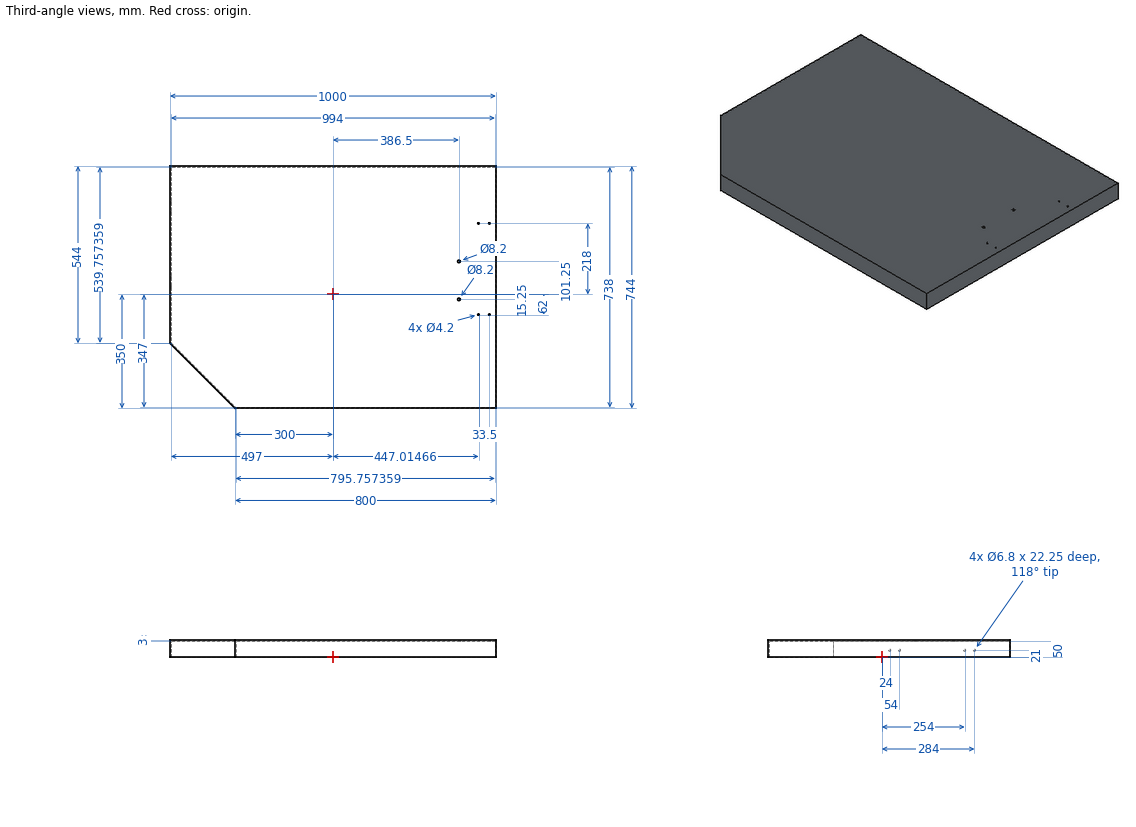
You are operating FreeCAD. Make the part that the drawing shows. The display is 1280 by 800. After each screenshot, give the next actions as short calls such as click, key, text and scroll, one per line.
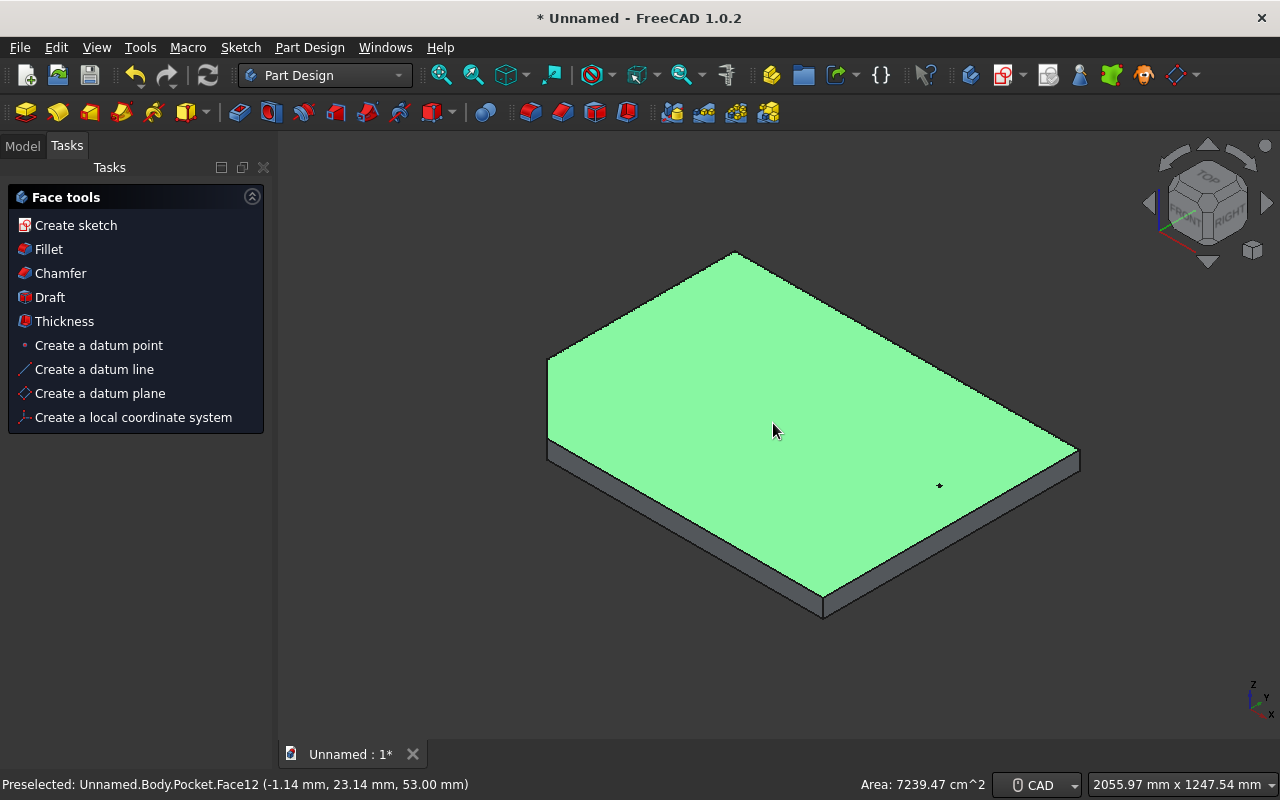
click(1004, 76)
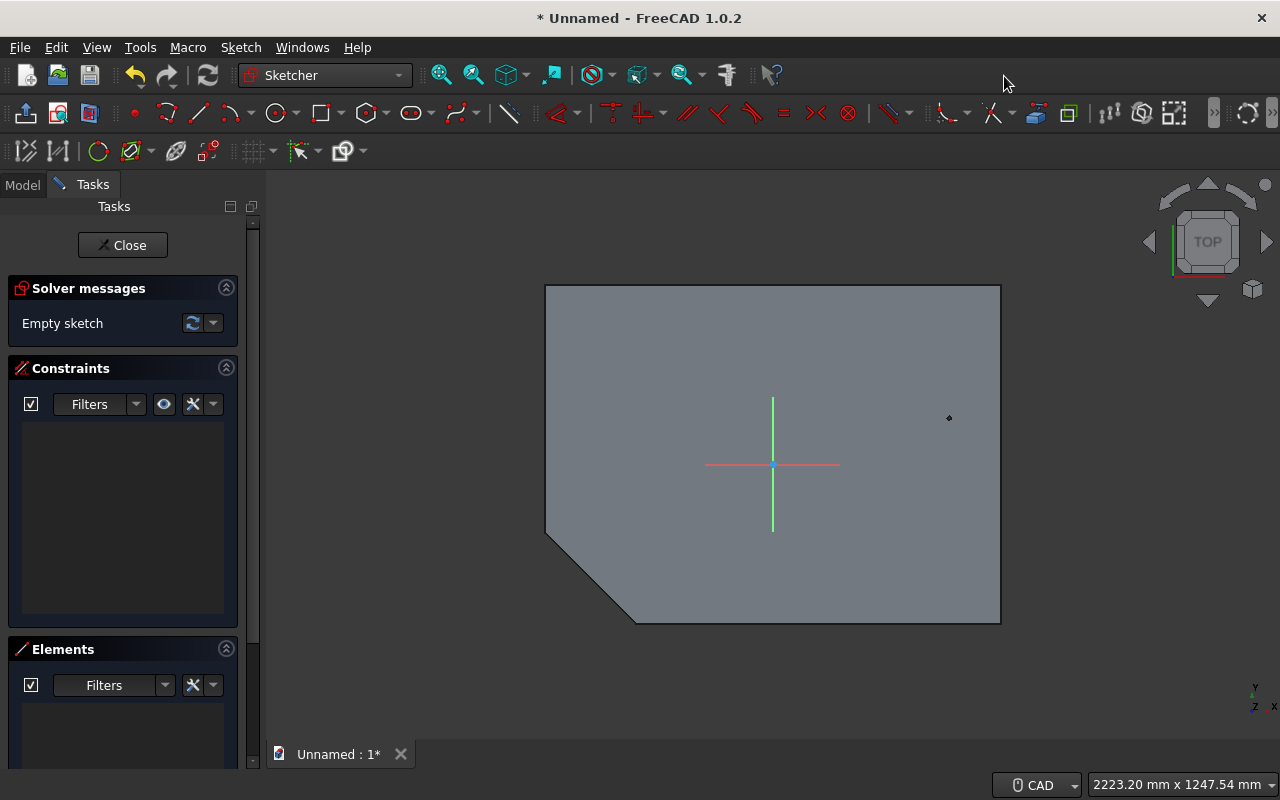
scroll(962, 472, up, 15)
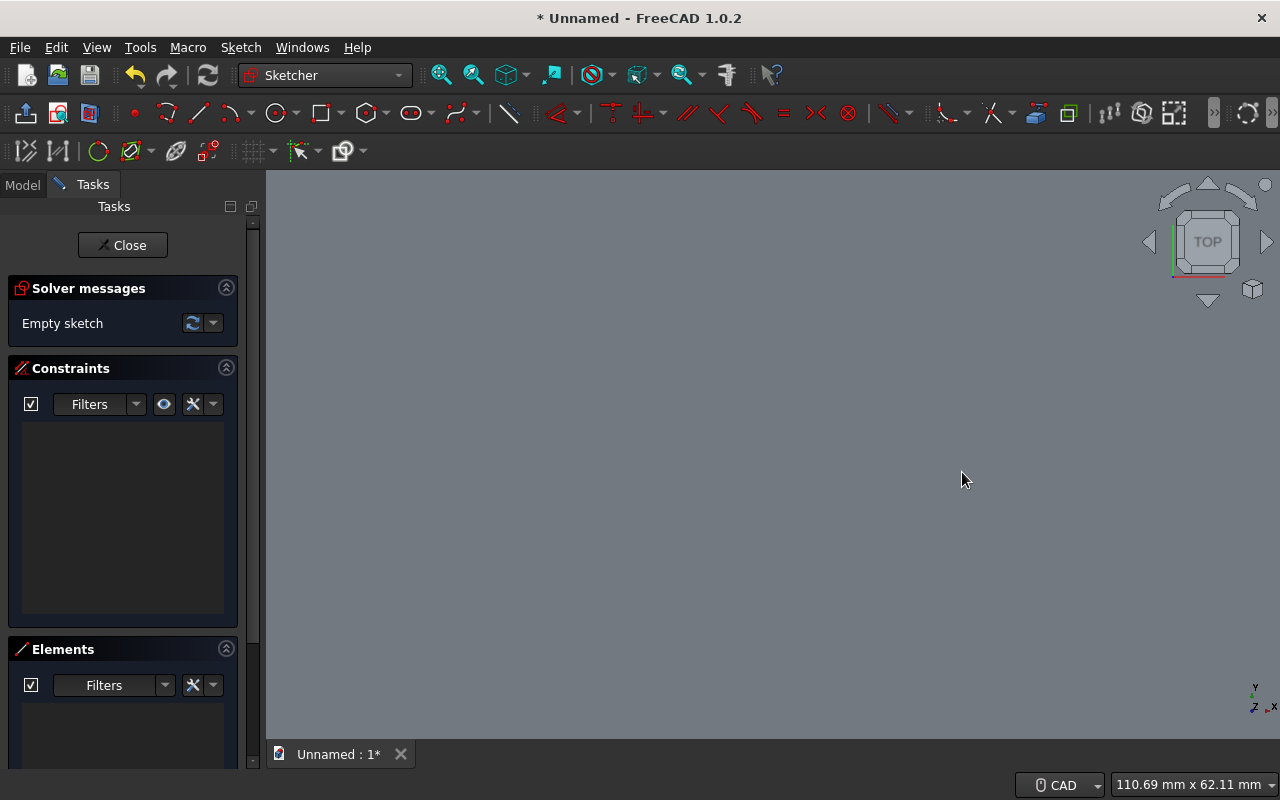
scroll(691, 451, up, 8)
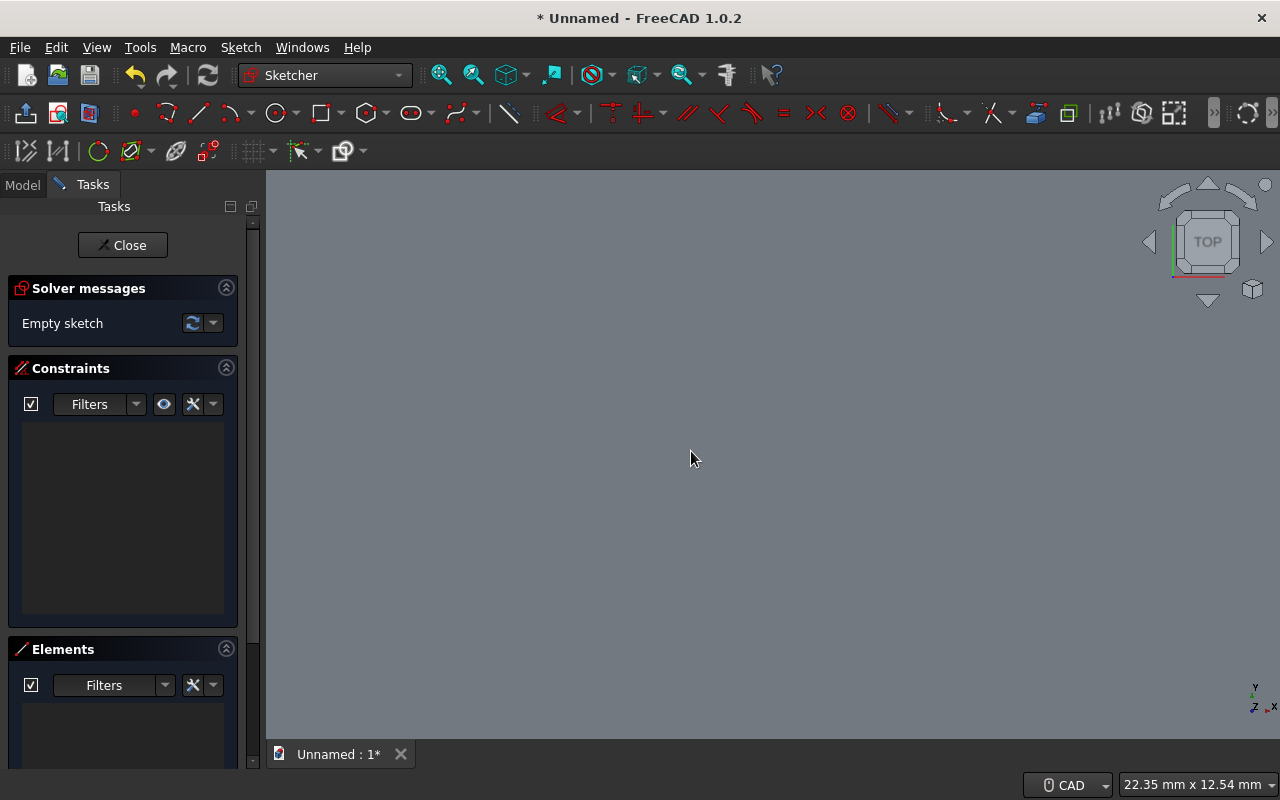
click(276, 114)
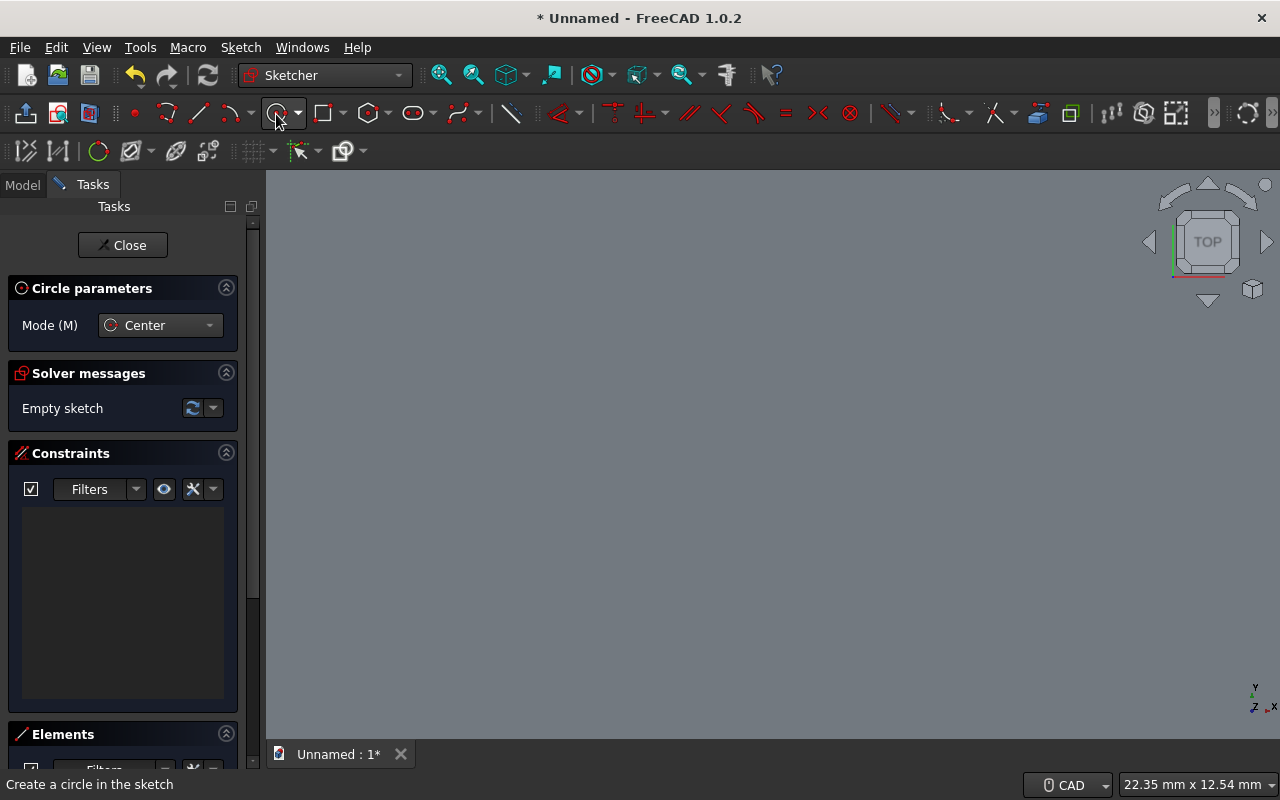
click(701, 452)
move(833, 320)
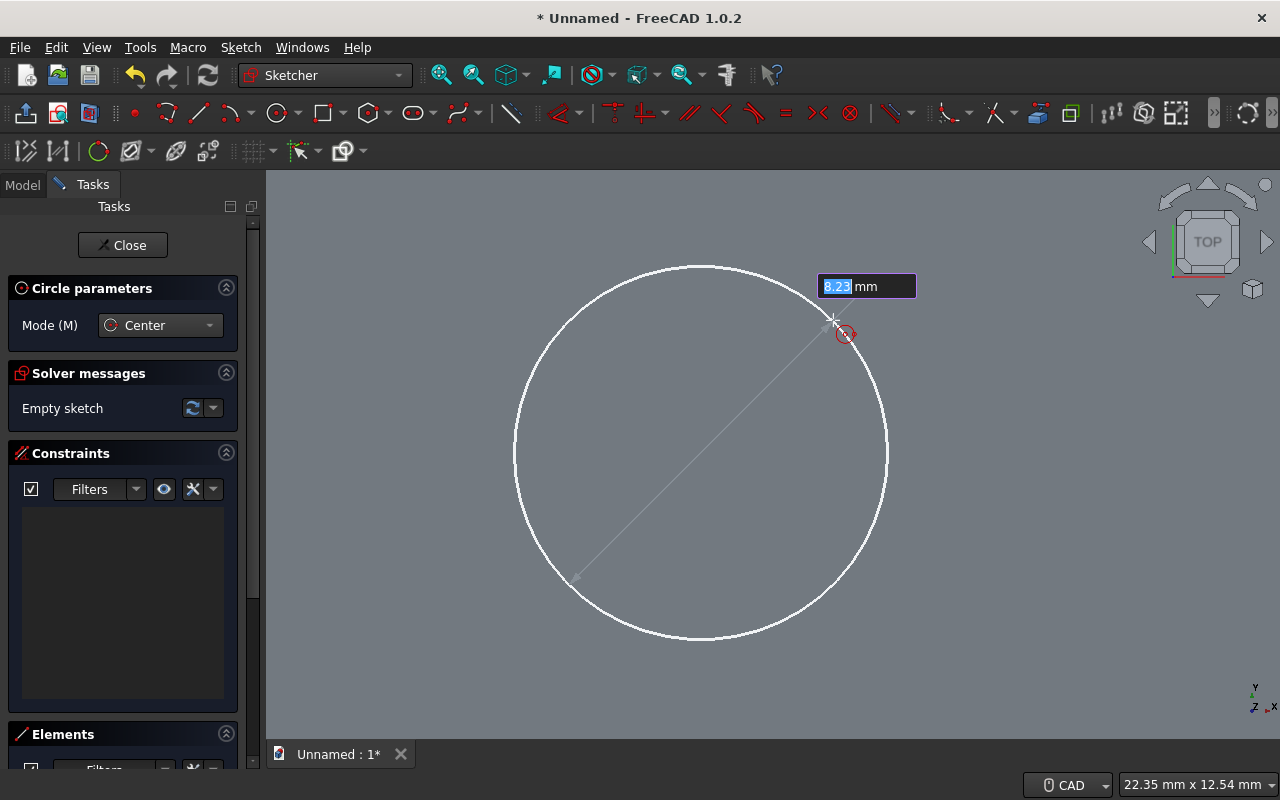
text(8.2)
key(Return)
key(Escape)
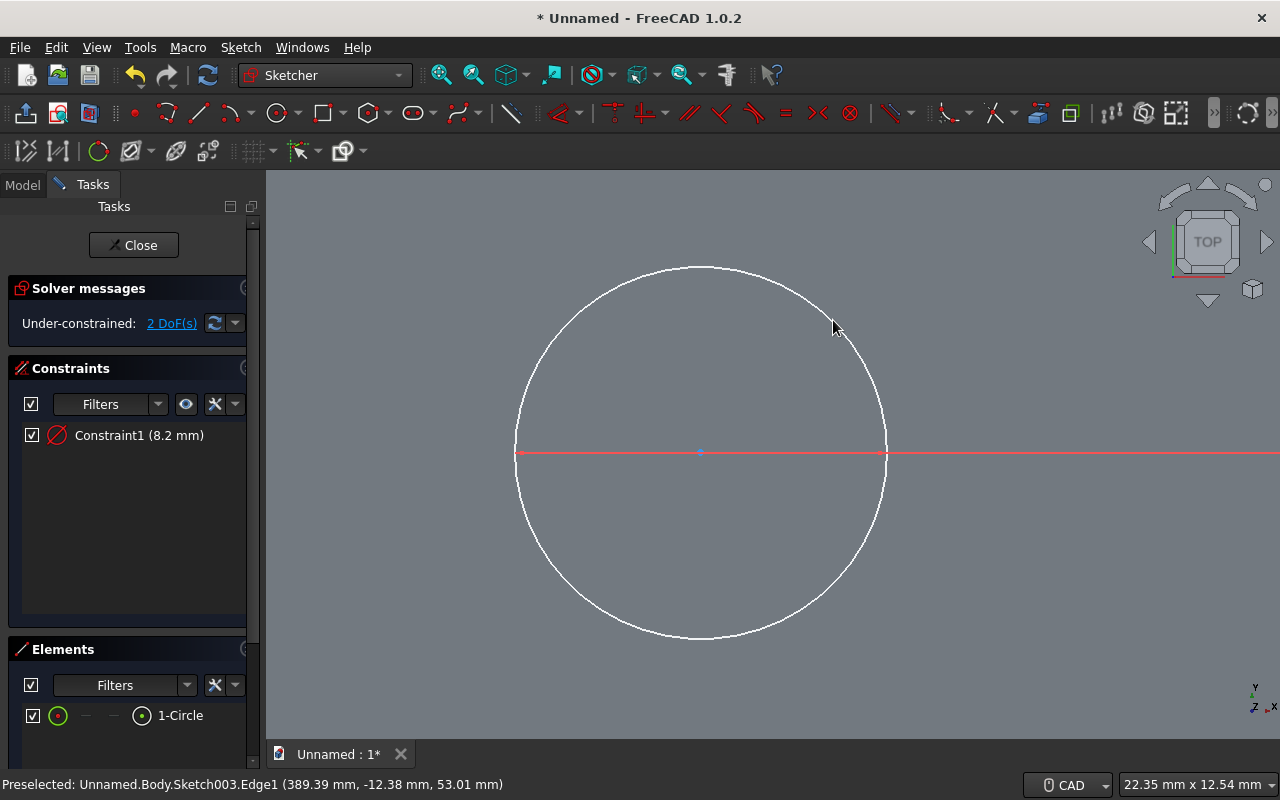
click(558, 114)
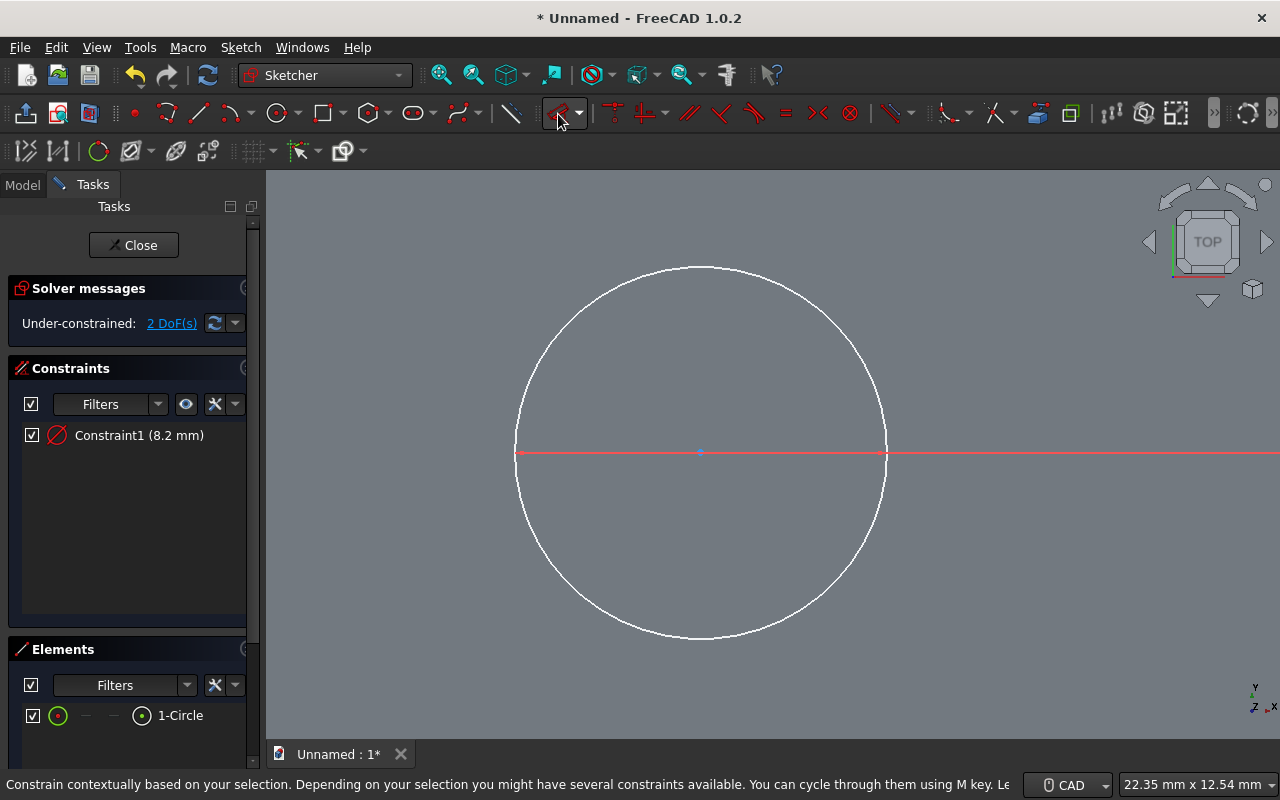
click(701, 453)
click(497, 487)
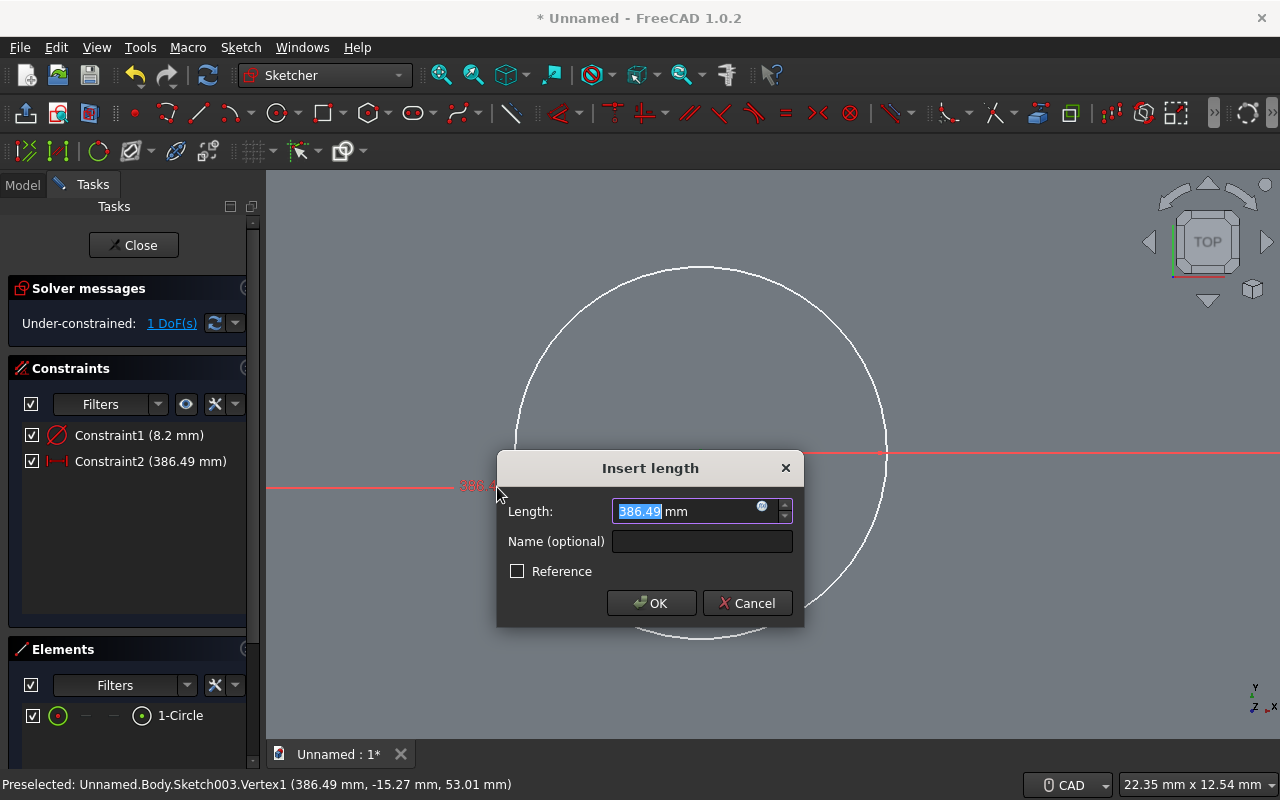
text(386.5)
key(Return)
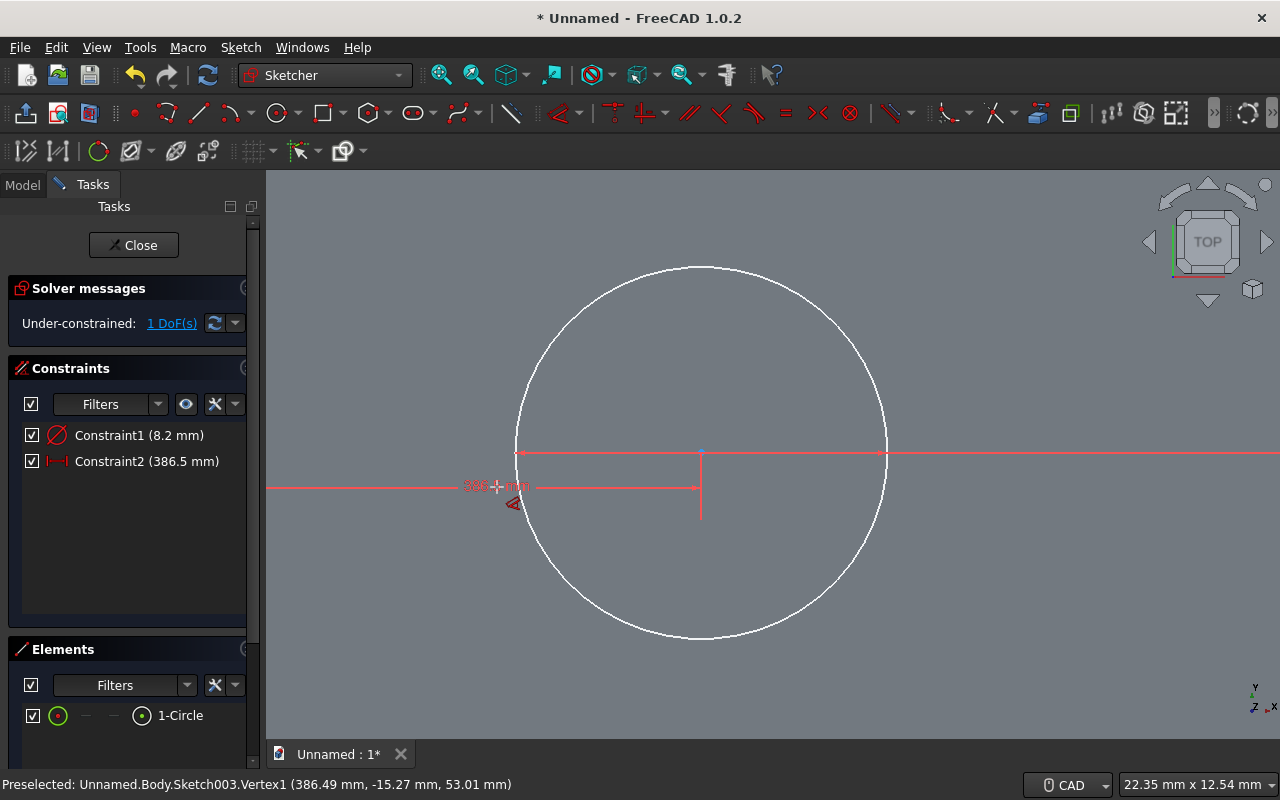
click(701, 453)
click(735, 325)